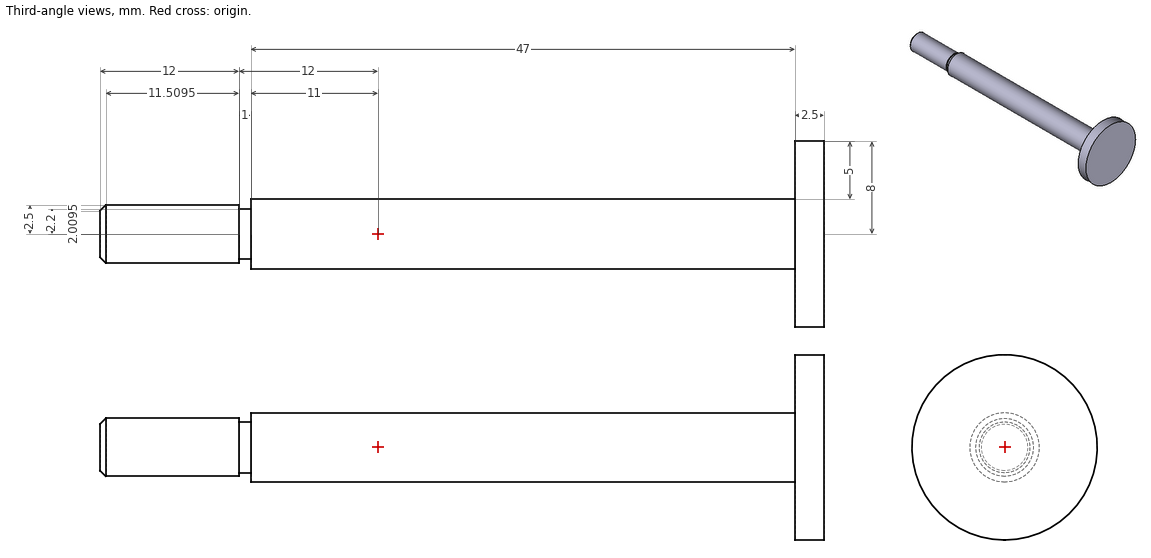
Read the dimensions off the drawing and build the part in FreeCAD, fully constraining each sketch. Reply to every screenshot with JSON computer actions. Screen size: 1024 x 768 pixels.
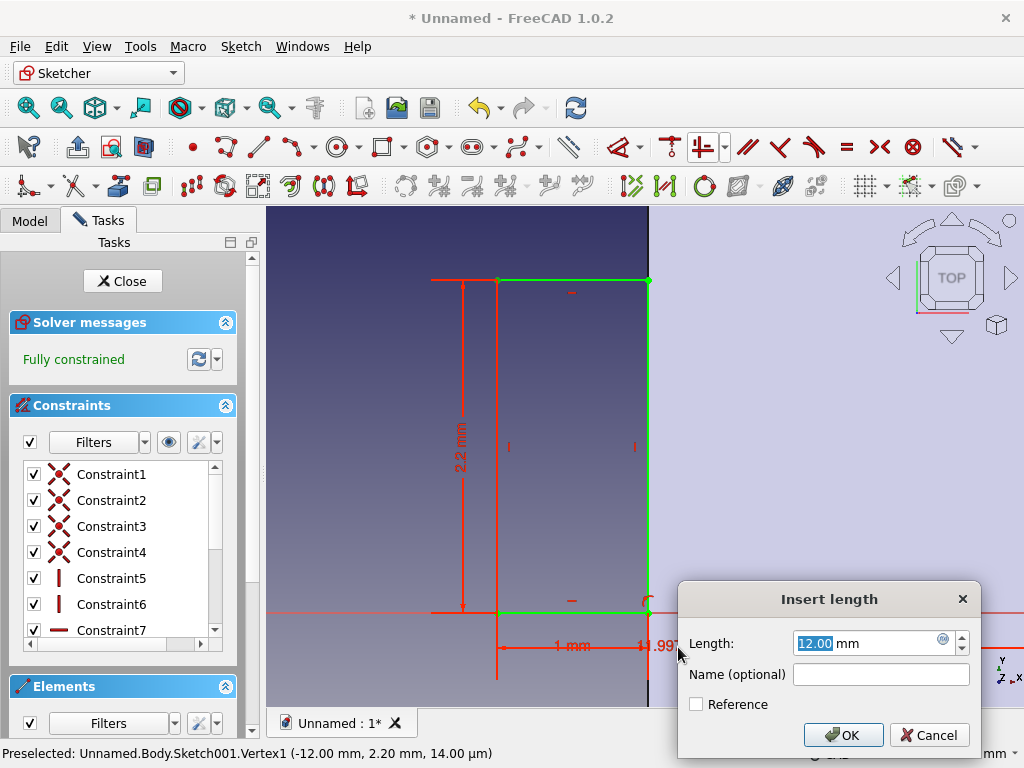
{"action": "type", "text": "12"}
{"action": "key", "text": "Return"}
{"action": "key", "text": "Escape"}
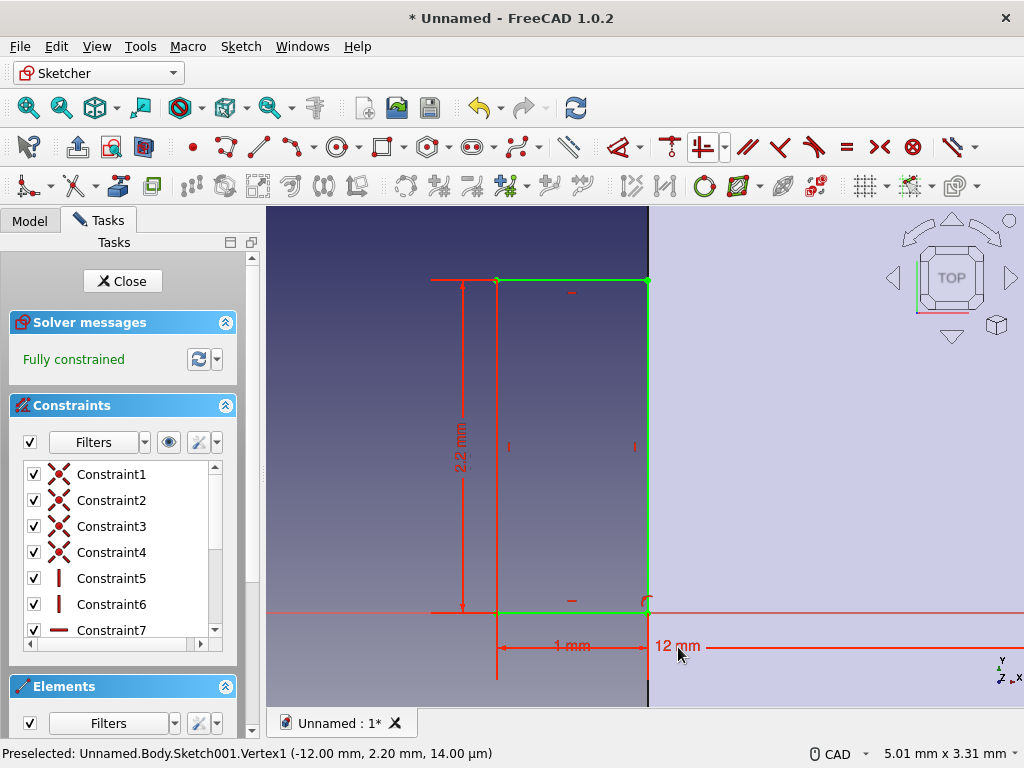
{"action": "left_click", "coordinate": [123, 281]}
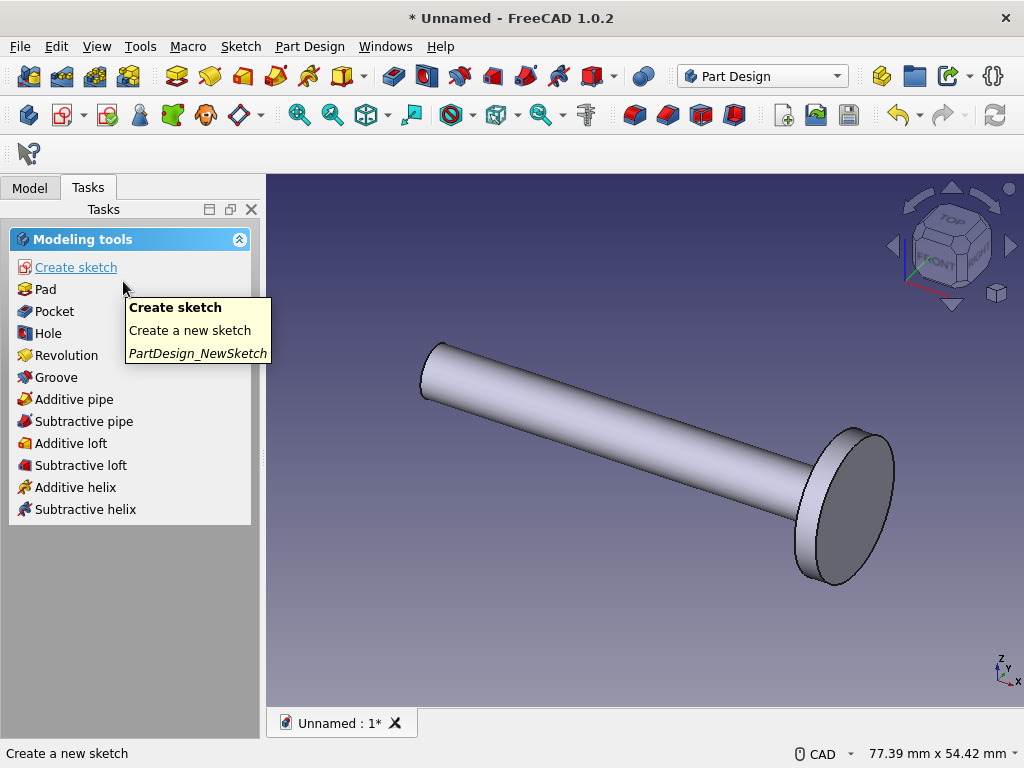
{"action": "left_click", "coordinate": [210, 76]}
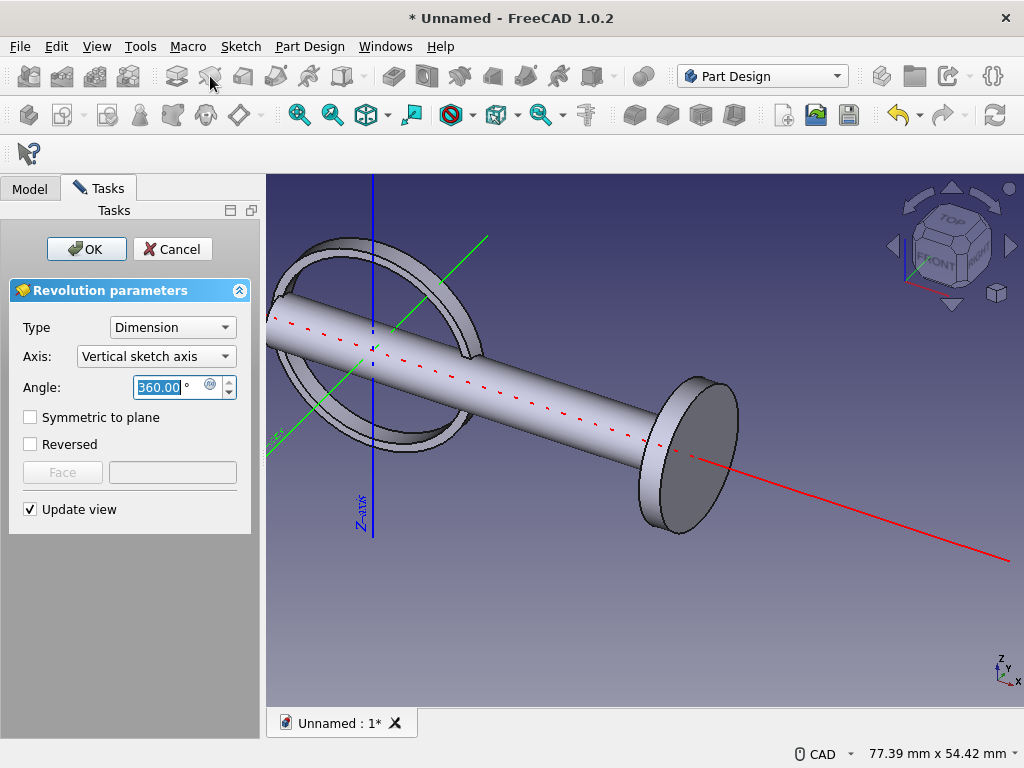
{"action": "left_click", "coordinate": [157, 356]}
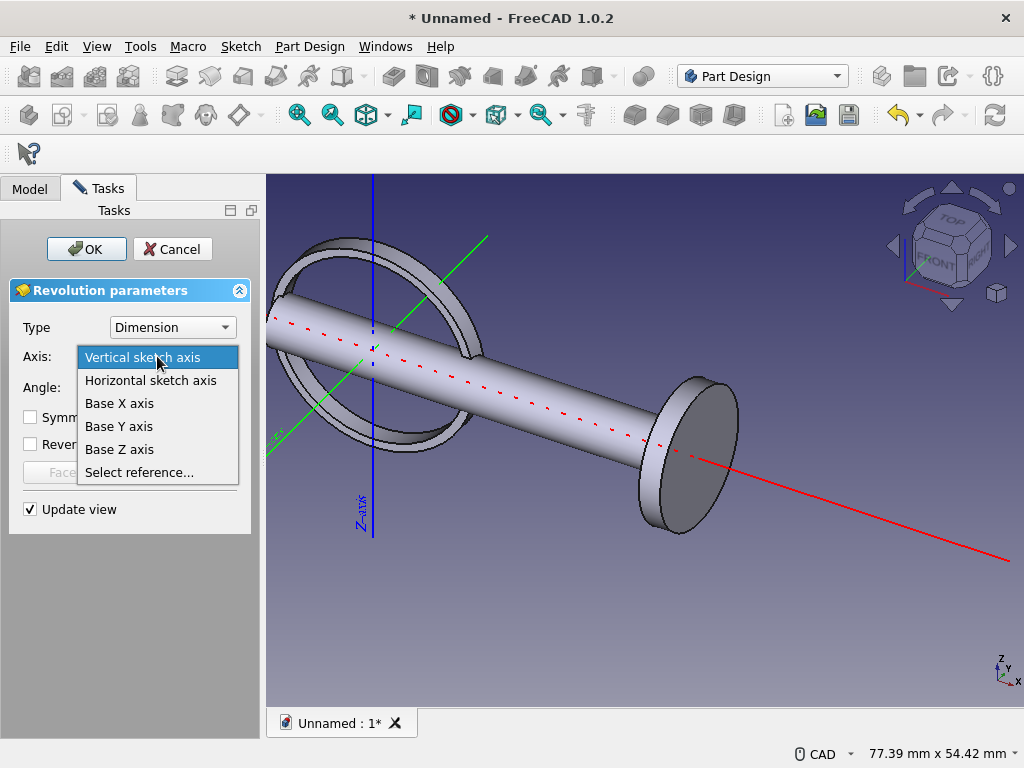
{"action": "left_click", "coordinate": [156, 380]}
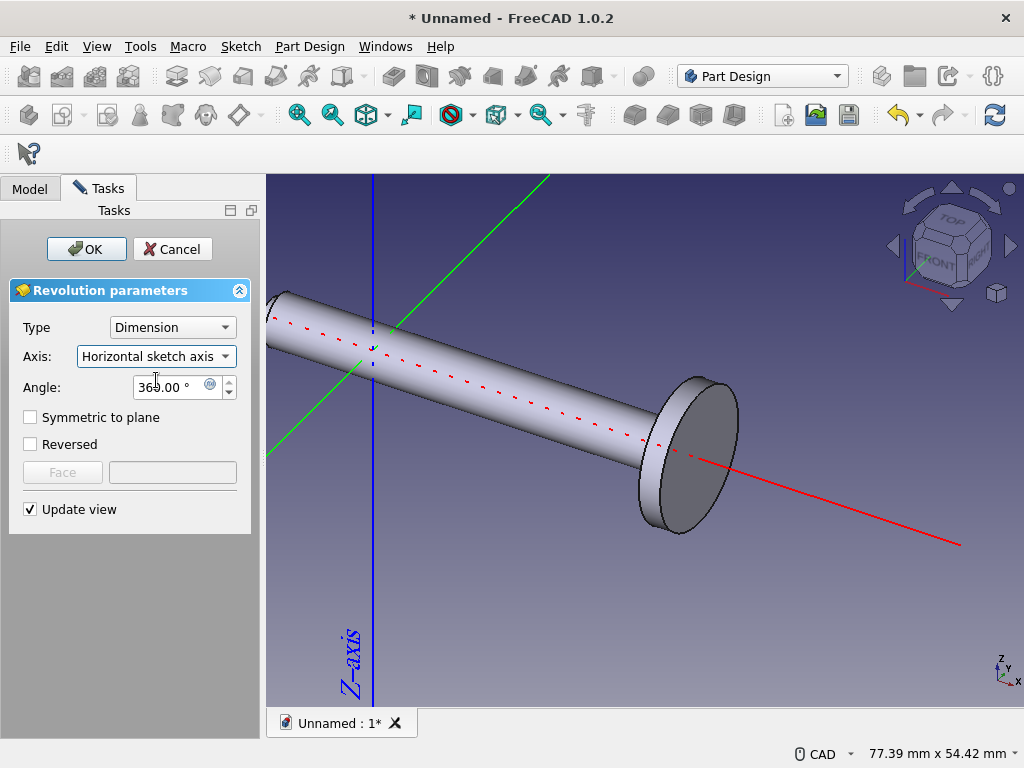
{"action": "left_click", "coordinate": [87, 249]}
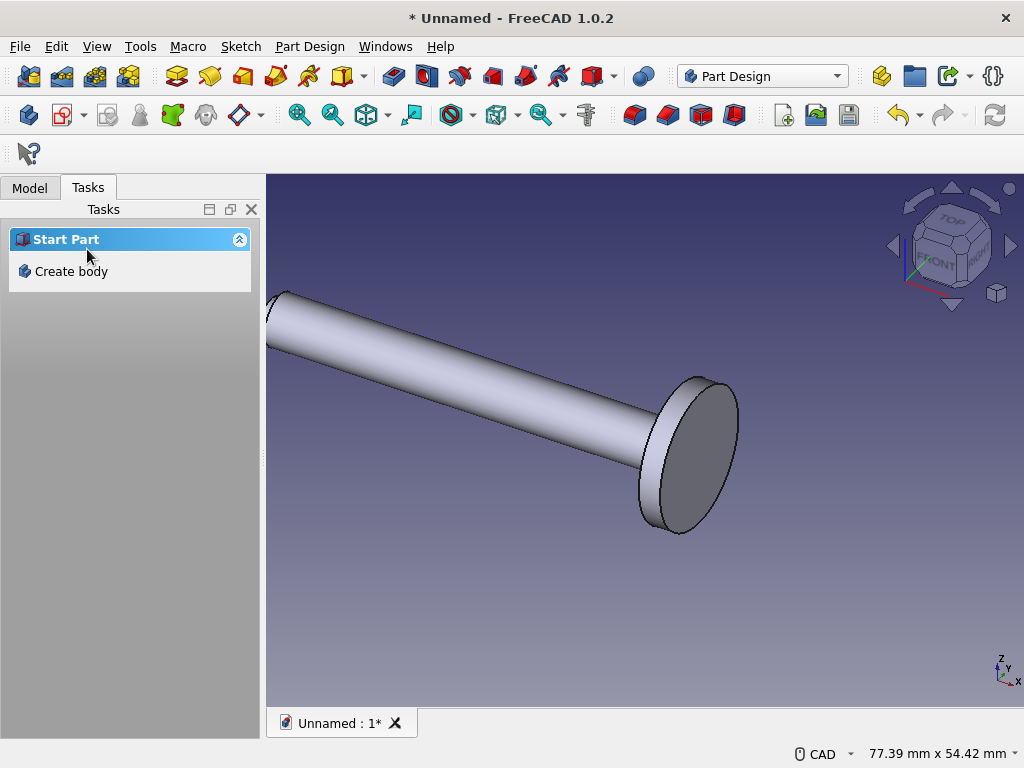
{"action": "left_click", "coordinate": [300, 116]}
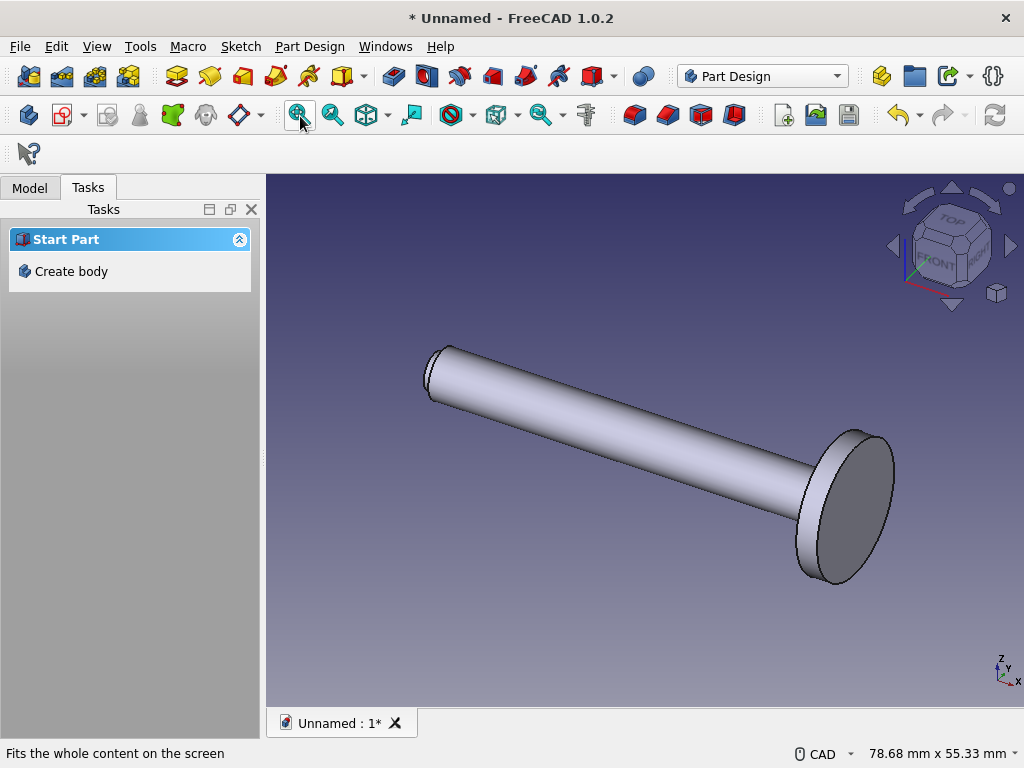
{"action": "left_click", "coordinate": [62, 116]}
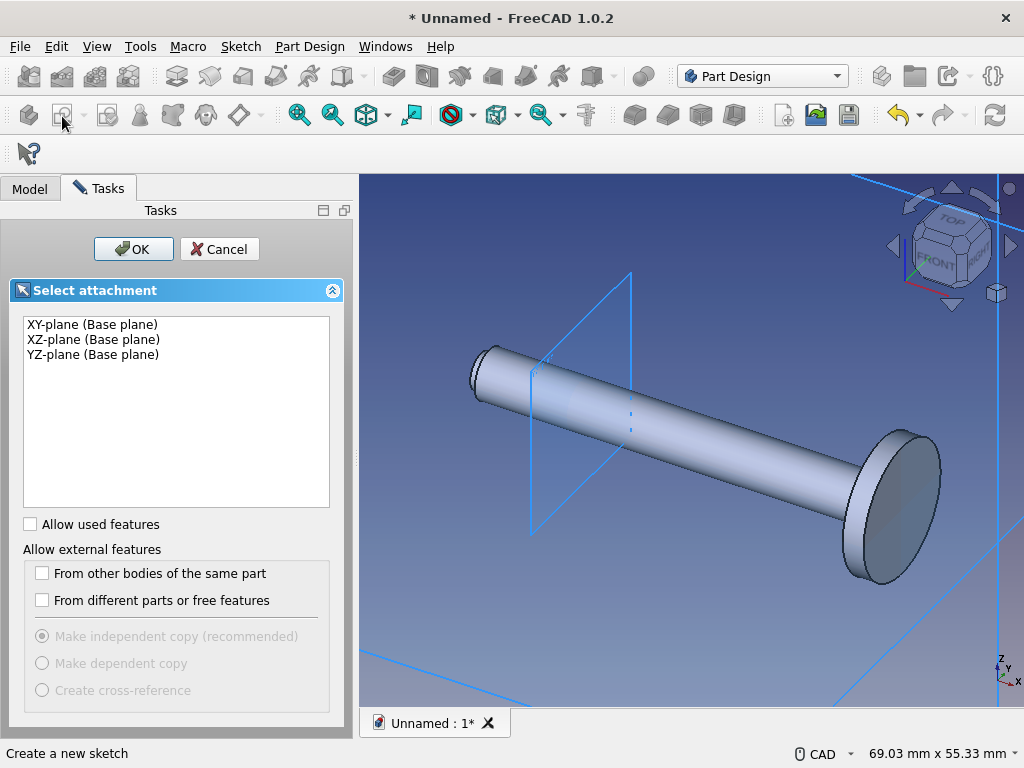
{"action": "left_click", "coordinate": [84, 324]}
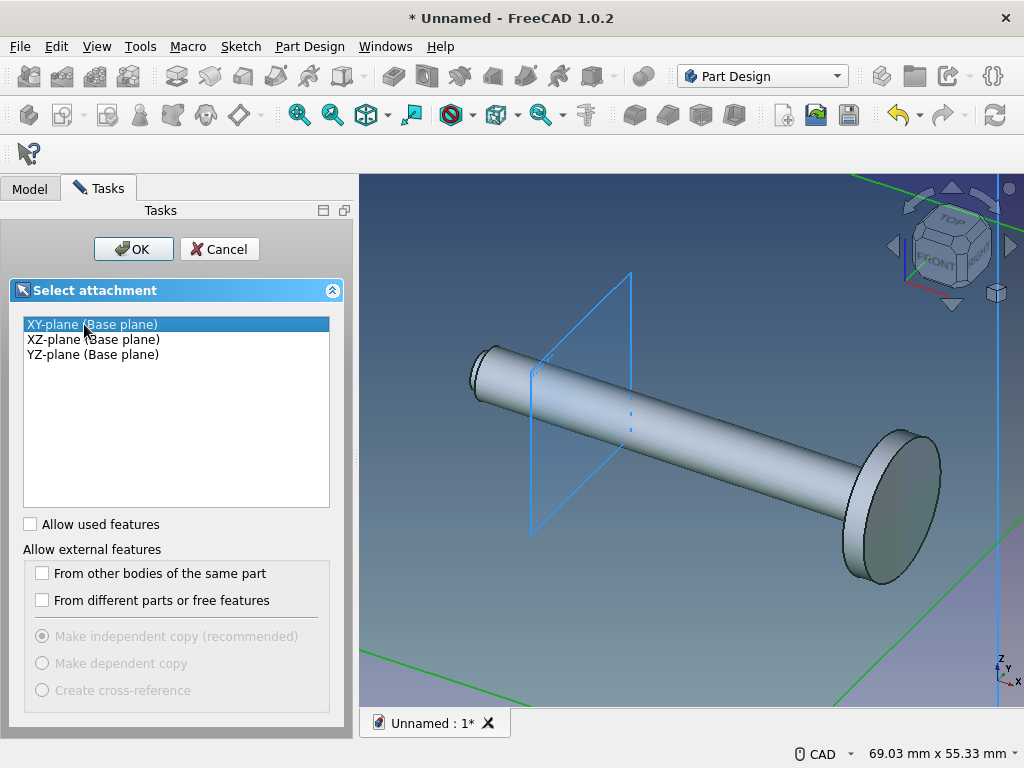
{"action": "left_click", "coordinate": [134, 249]}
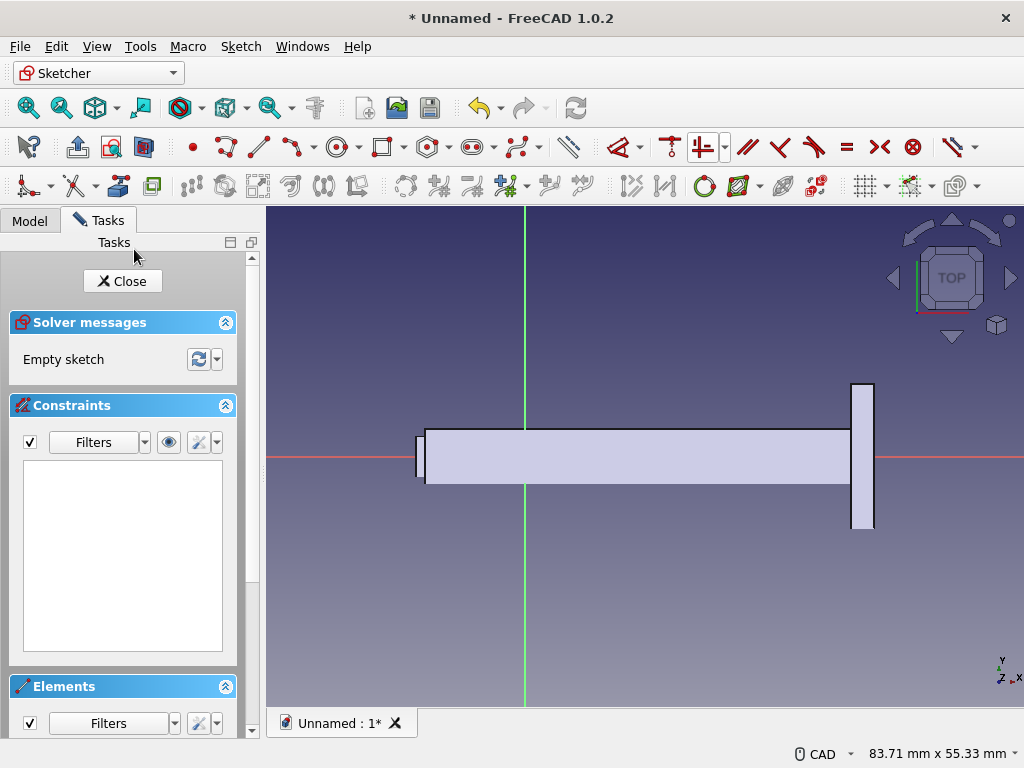
{"action": "left_click", "coordinate": [144, 148]}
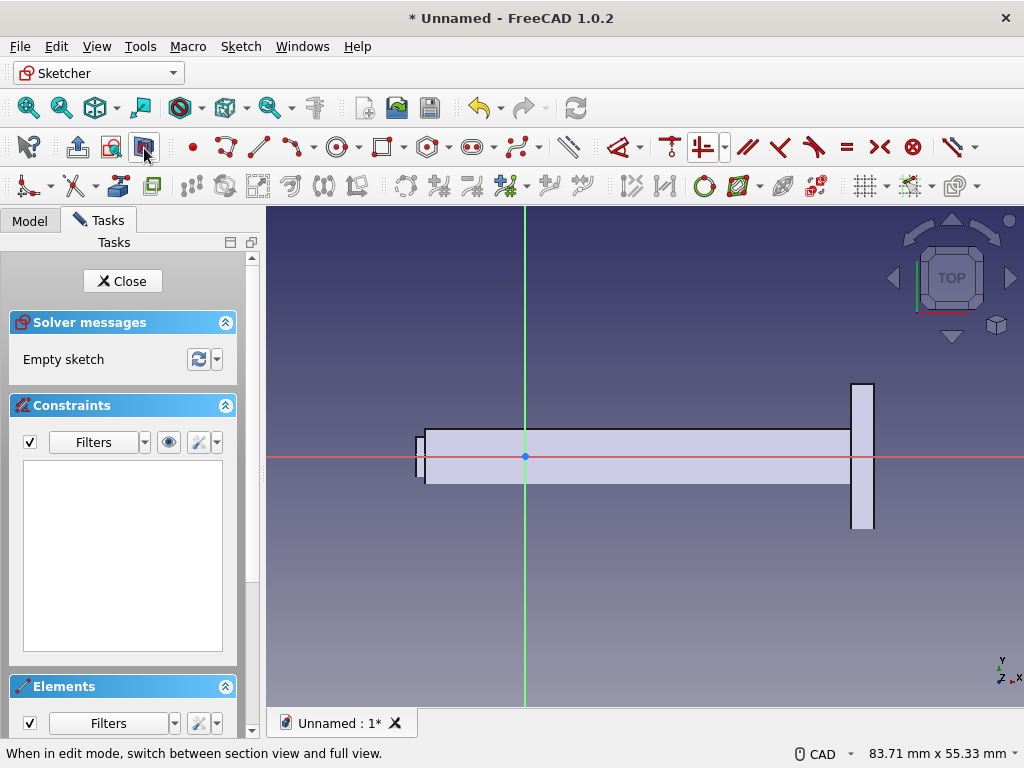
{"action": "scroll", "coordinate": [576, 456], "scroll_direction": "down", "scroll_amount": 5}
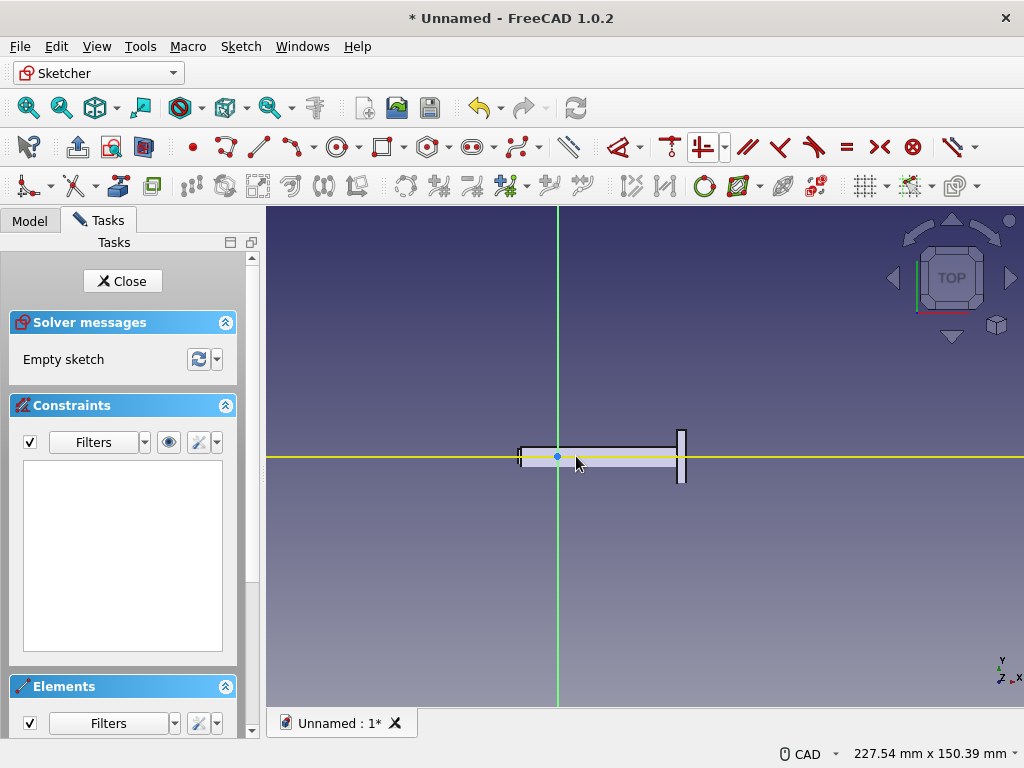
{"action": "scroll", "coordinate": [503, 451], "scroll_direction": "up", "scroll_amount": 8}